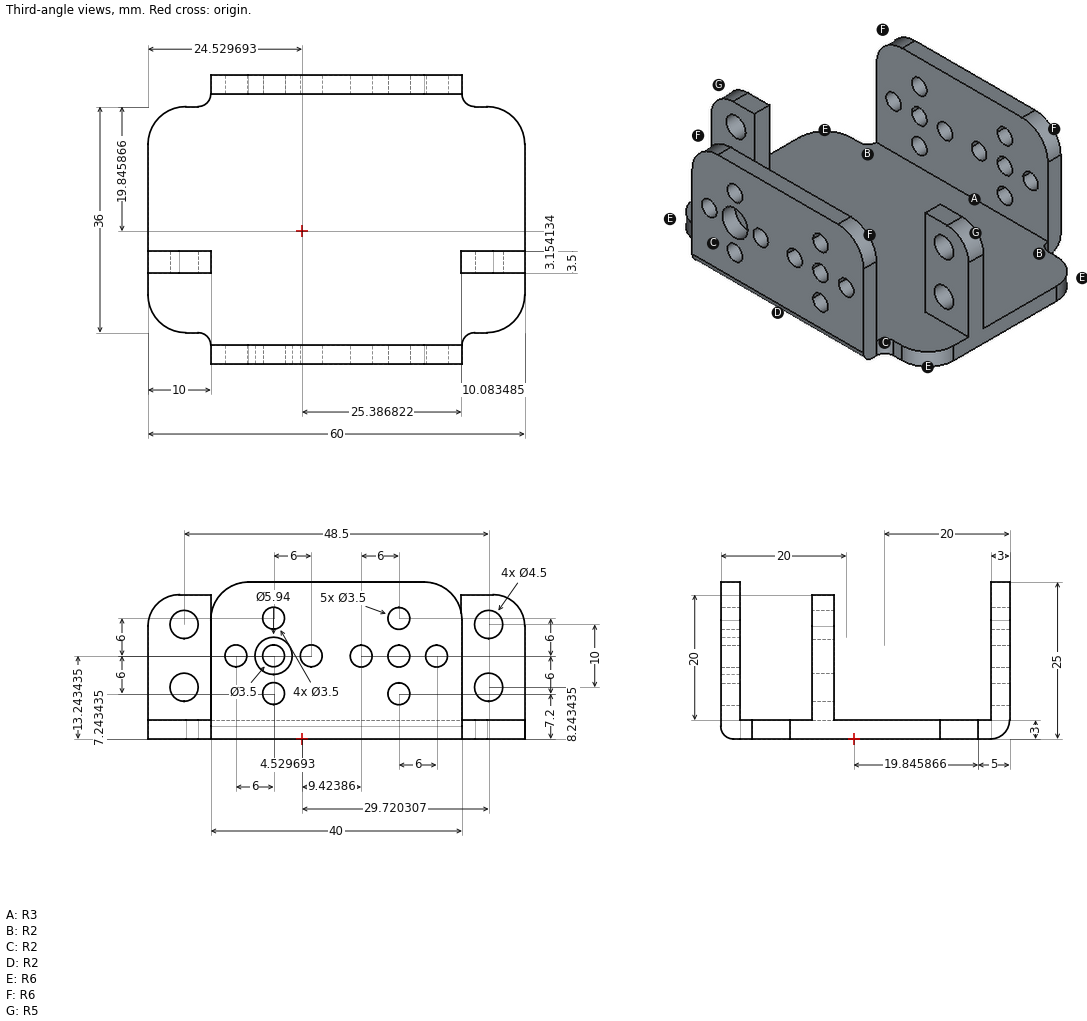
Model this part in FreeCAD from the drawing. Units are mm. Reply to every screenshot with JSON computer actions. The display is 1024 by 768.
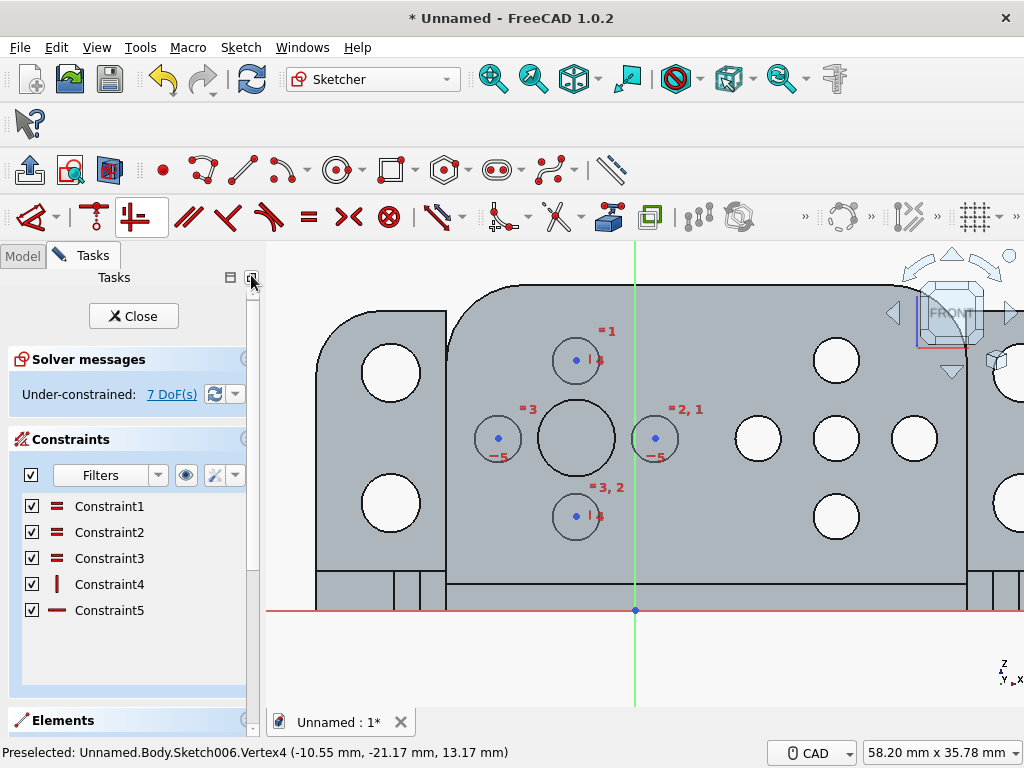
{"action": "left_click", "coordinate": [32, 218]}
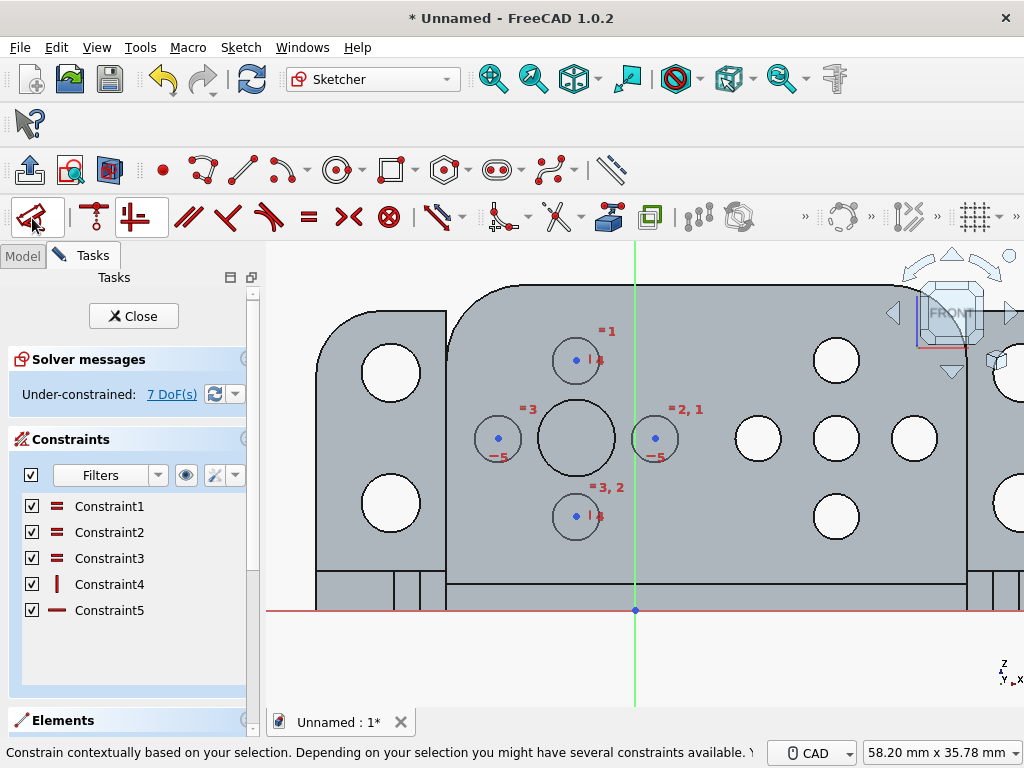
{"action": "left_click", "coordinate": [592, 344]}
{"action": "left_click", "coordinate": [614, 321]}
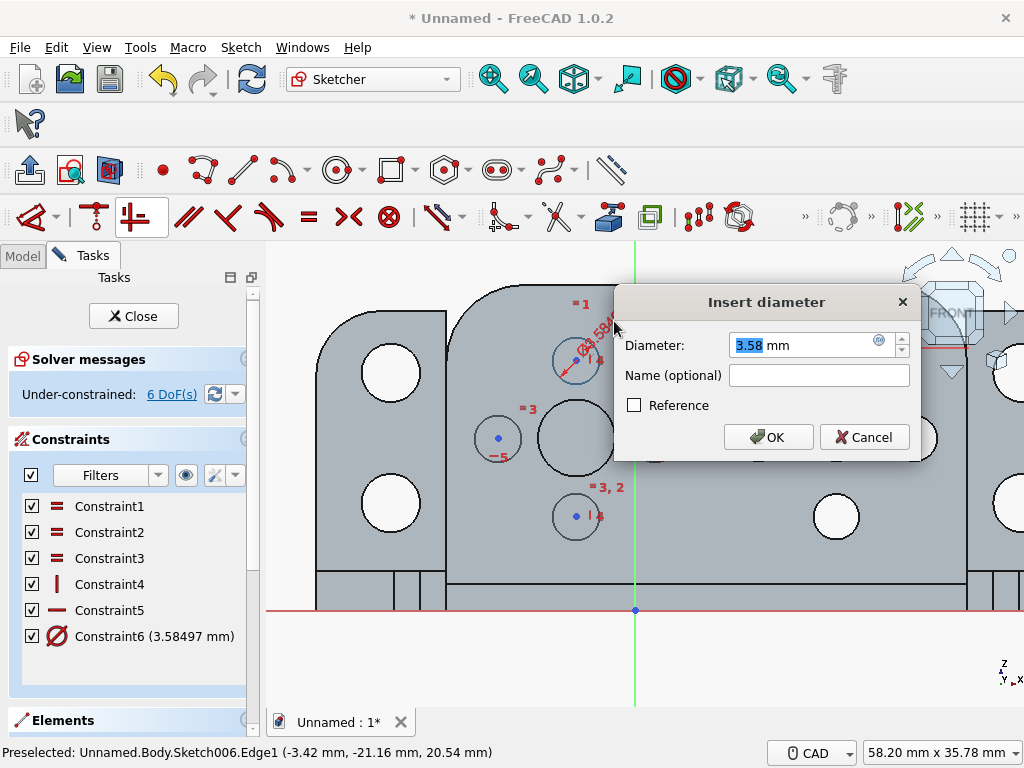
{"action": "type", "text": "3.5"}
{"action": "key", "text": "Return"}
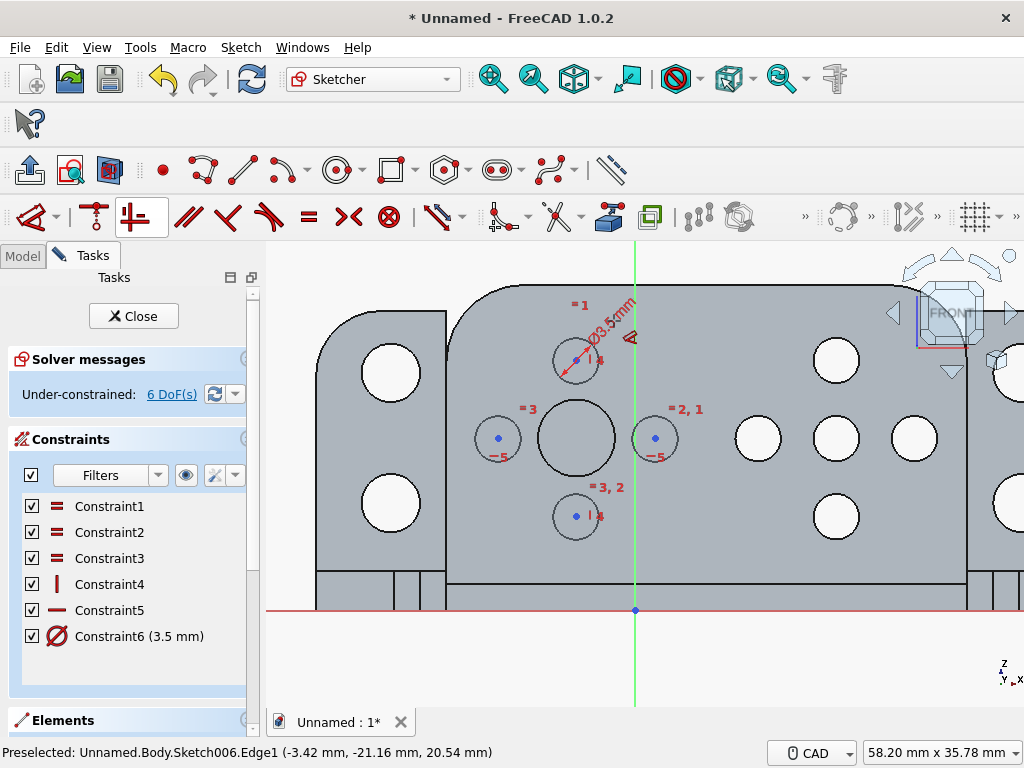
{"action": "left_click", "coordinate": [576, 361]}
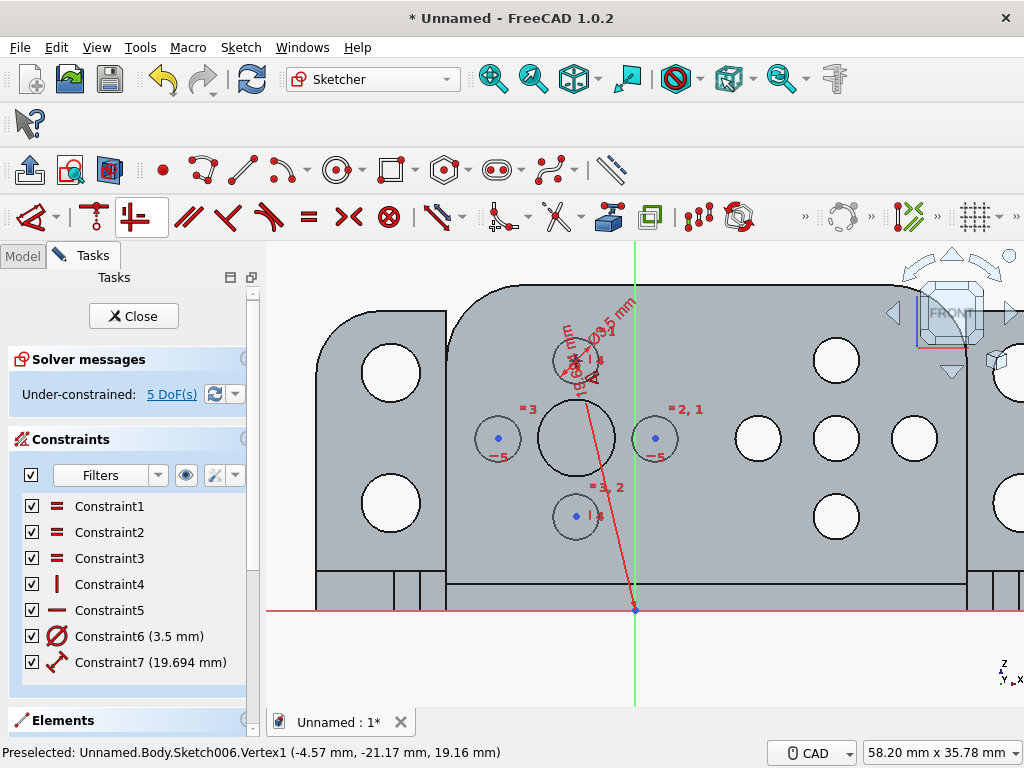
{"action": "left_click", "coordinate": [655, 439]}
{"action": "left_click", "coordinate": [615, 473]}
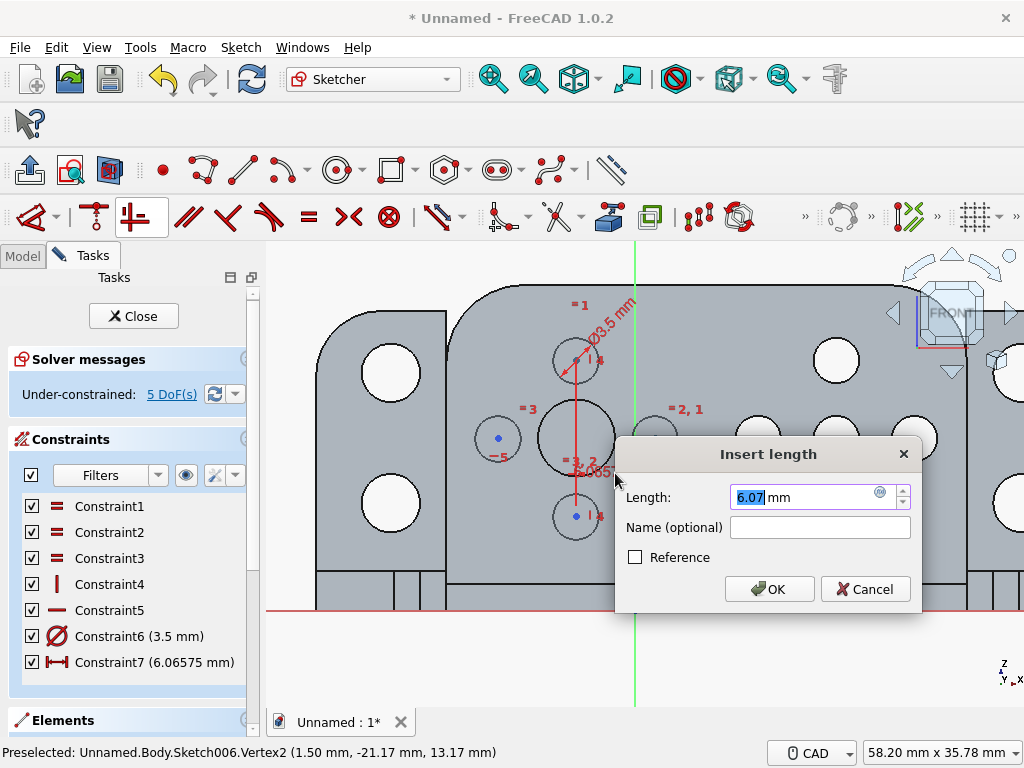
{"action": "type", "text": "6"}
{"action": "key", "text": "Return"}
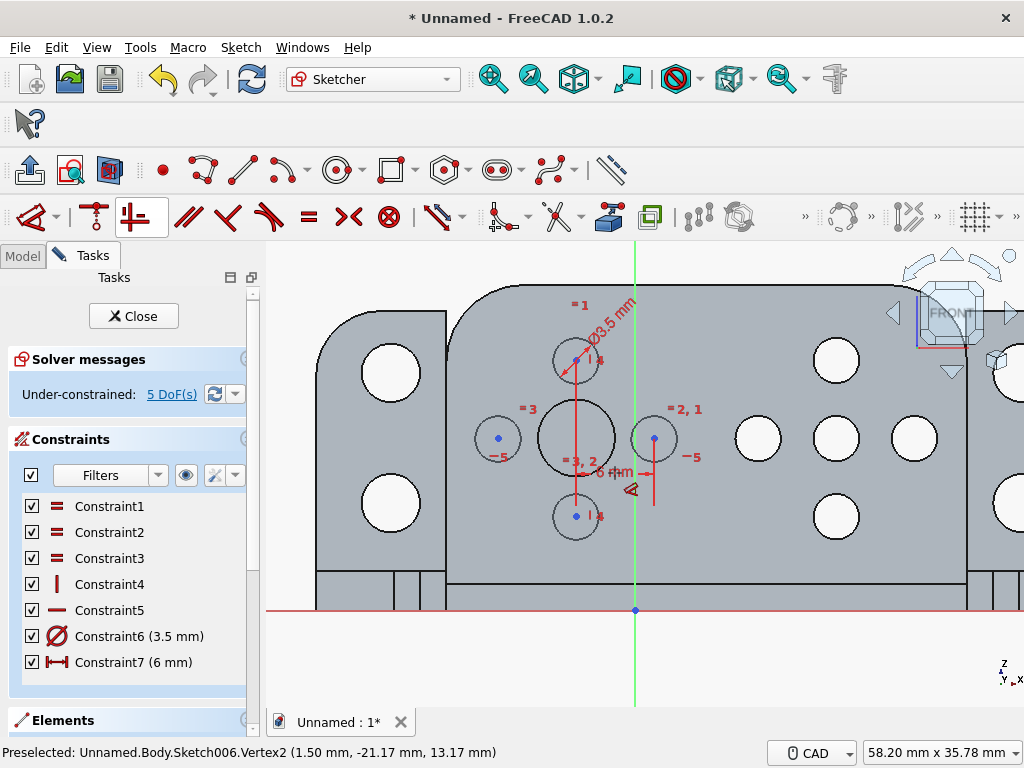
{"action": "left_click", "coordinate": [576, 361]}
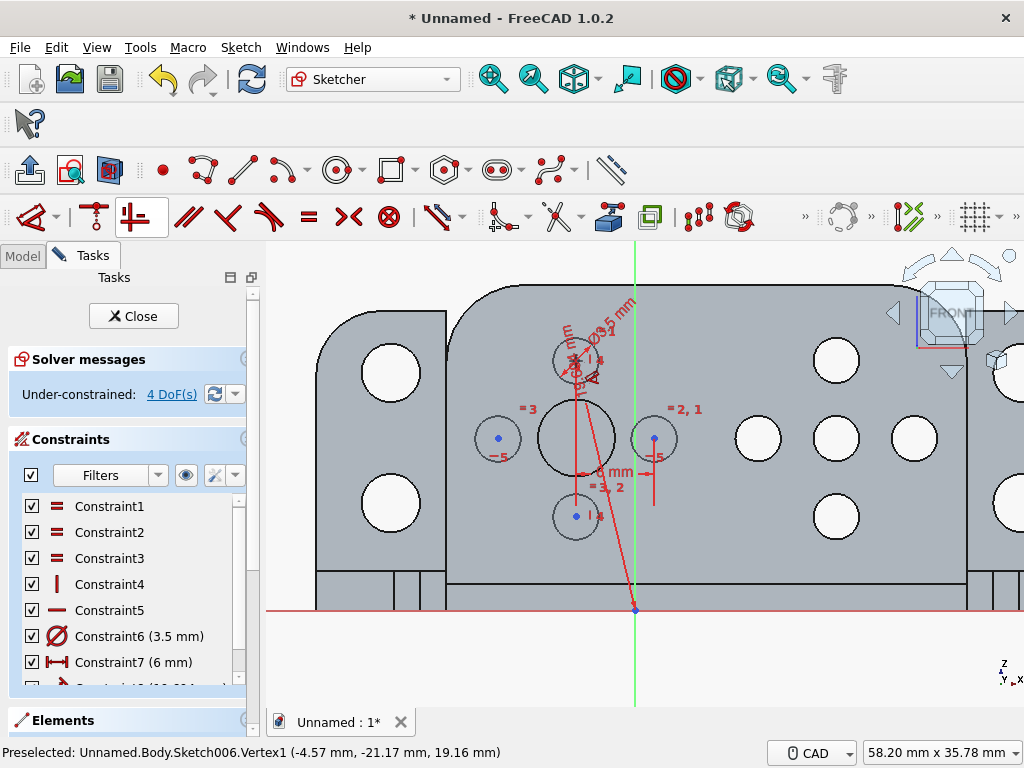
{"action": "left_click", "coordinate": [654, 439]}
{"action": "left_click", "coordinate": [688, 400]}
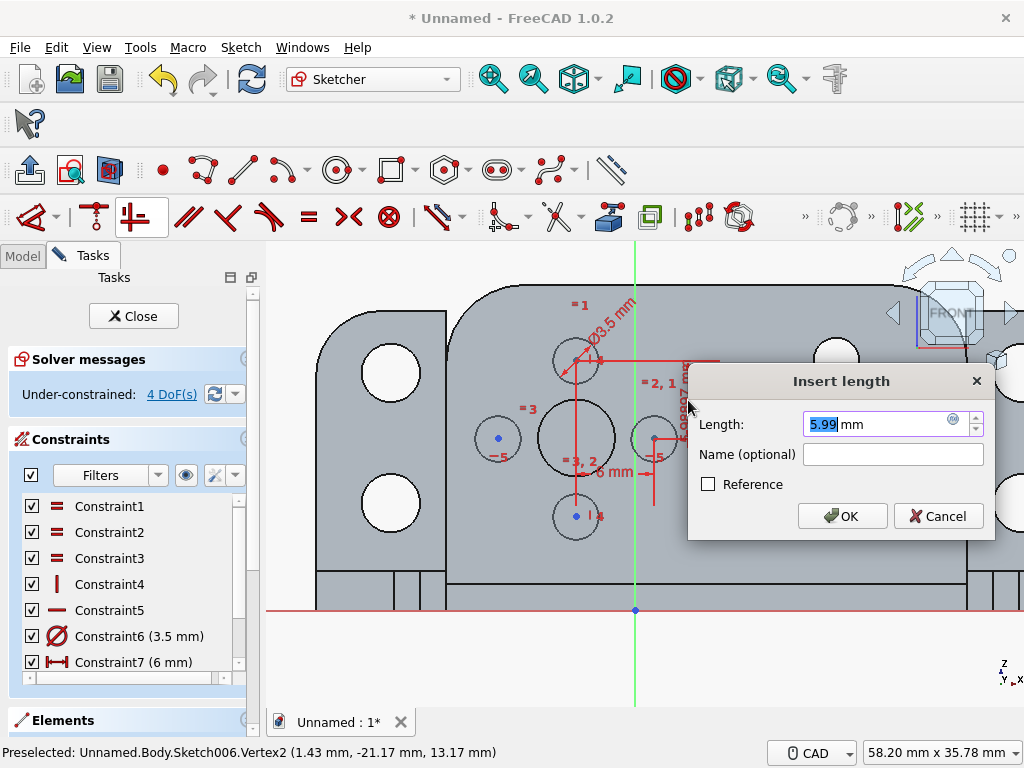
{"action": "type", "text": "6"}
{"action": "key", "text": "Return"}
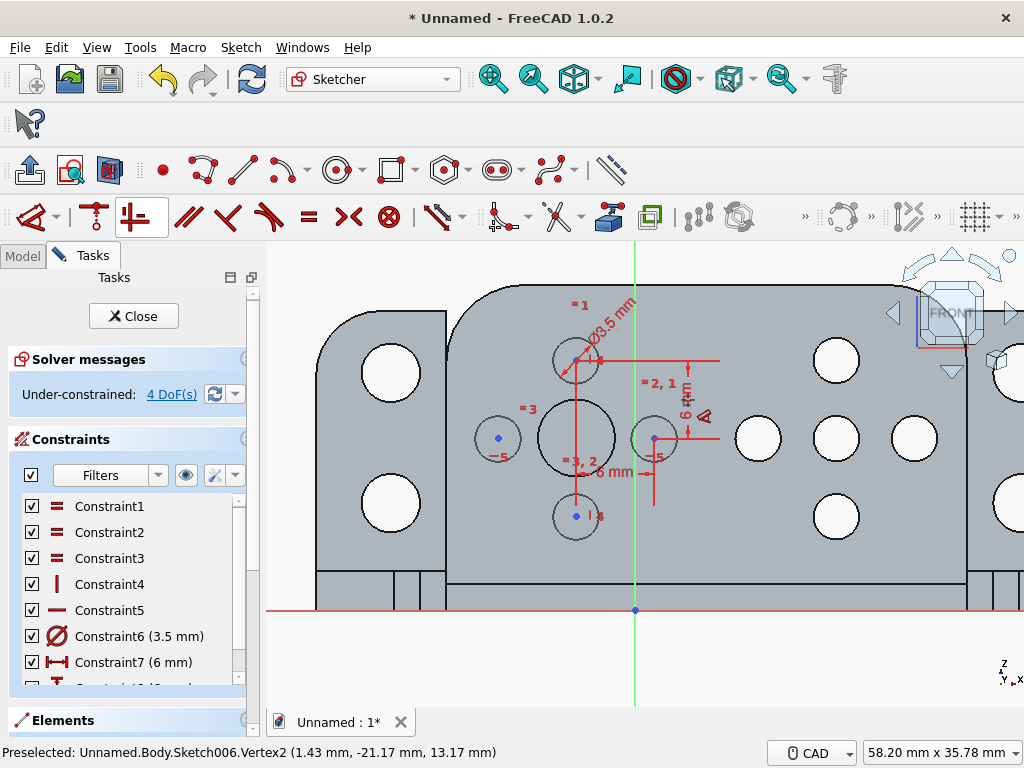
{"action": "left_click", "coordinate": [654, 439]}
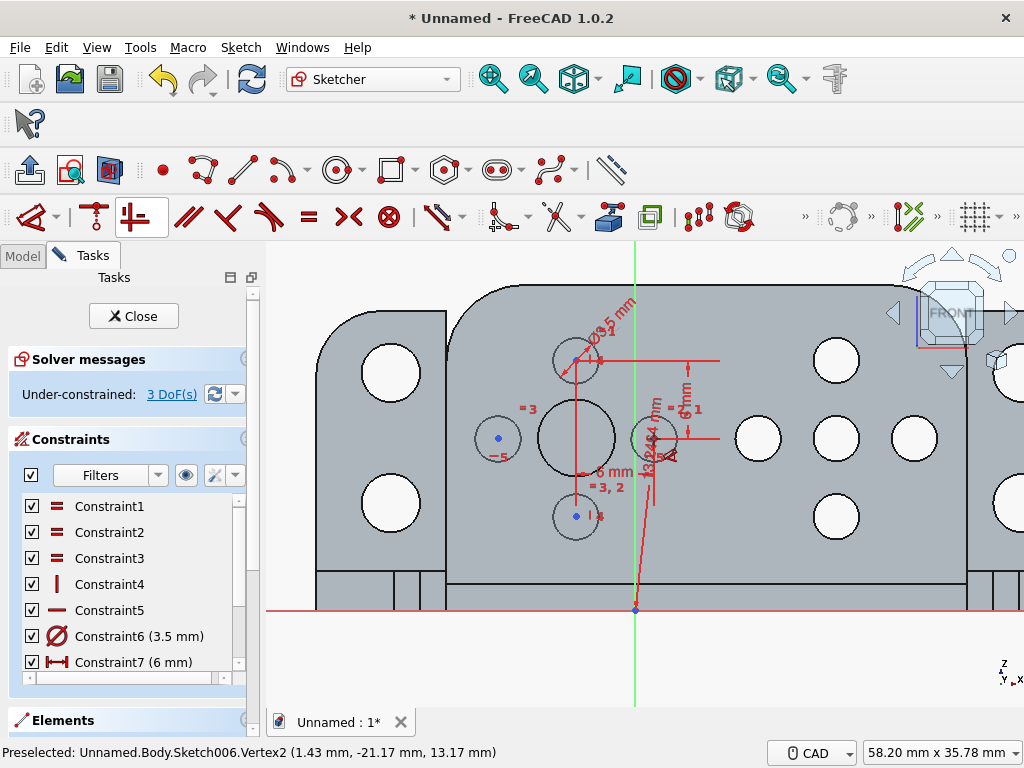
{"action": "left_click", "coordinate": [576, 517]}
{"action": "left_click", "coordinate": [688, 478]}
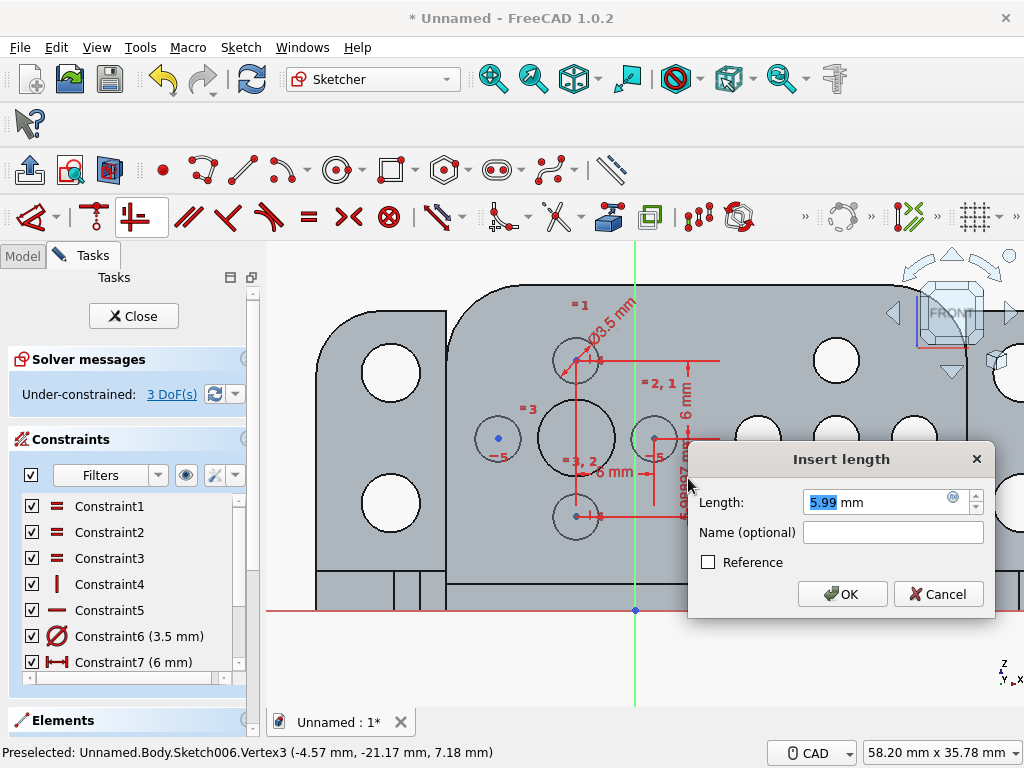
{"action": "type", "text": "6"}
{"action": "key", "text": "Return"}